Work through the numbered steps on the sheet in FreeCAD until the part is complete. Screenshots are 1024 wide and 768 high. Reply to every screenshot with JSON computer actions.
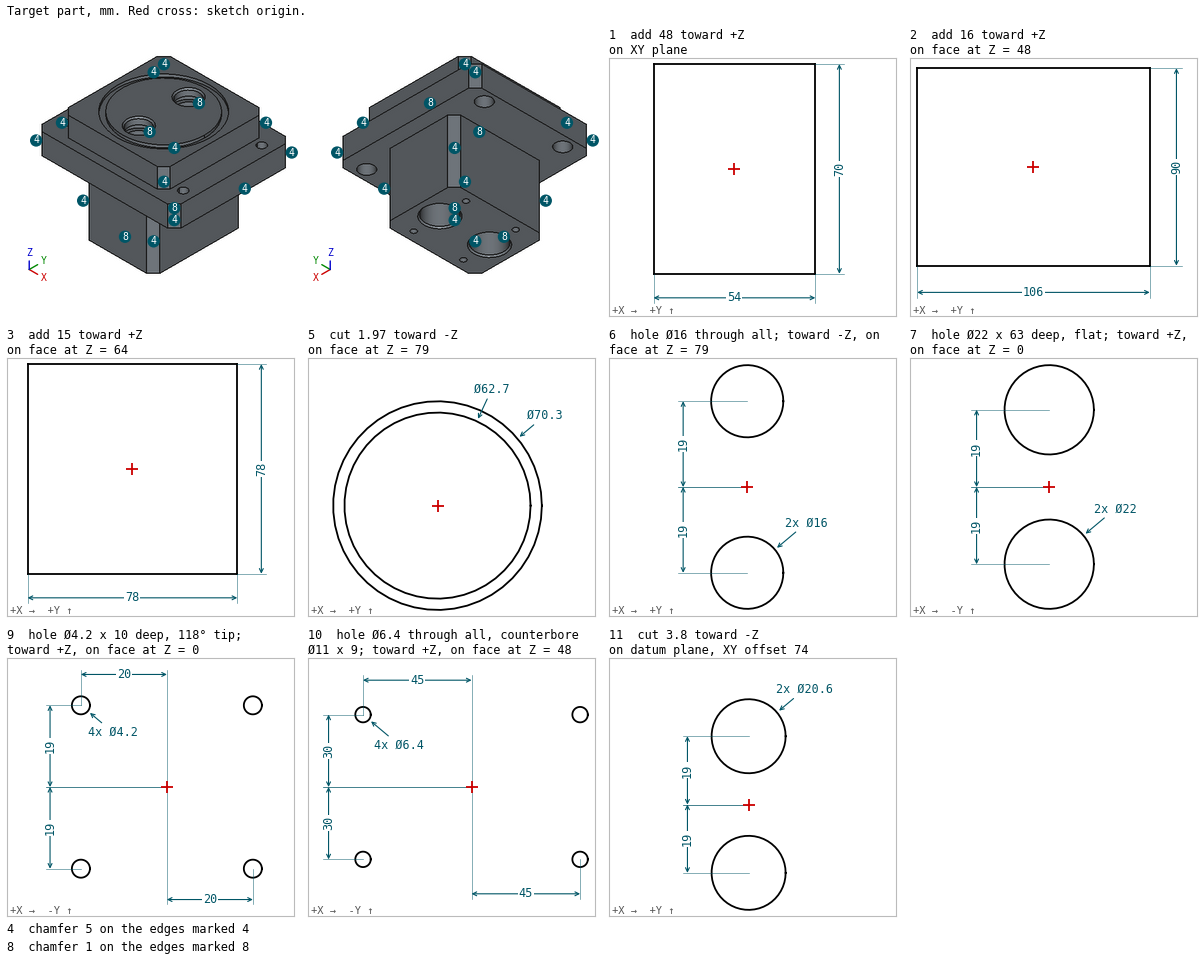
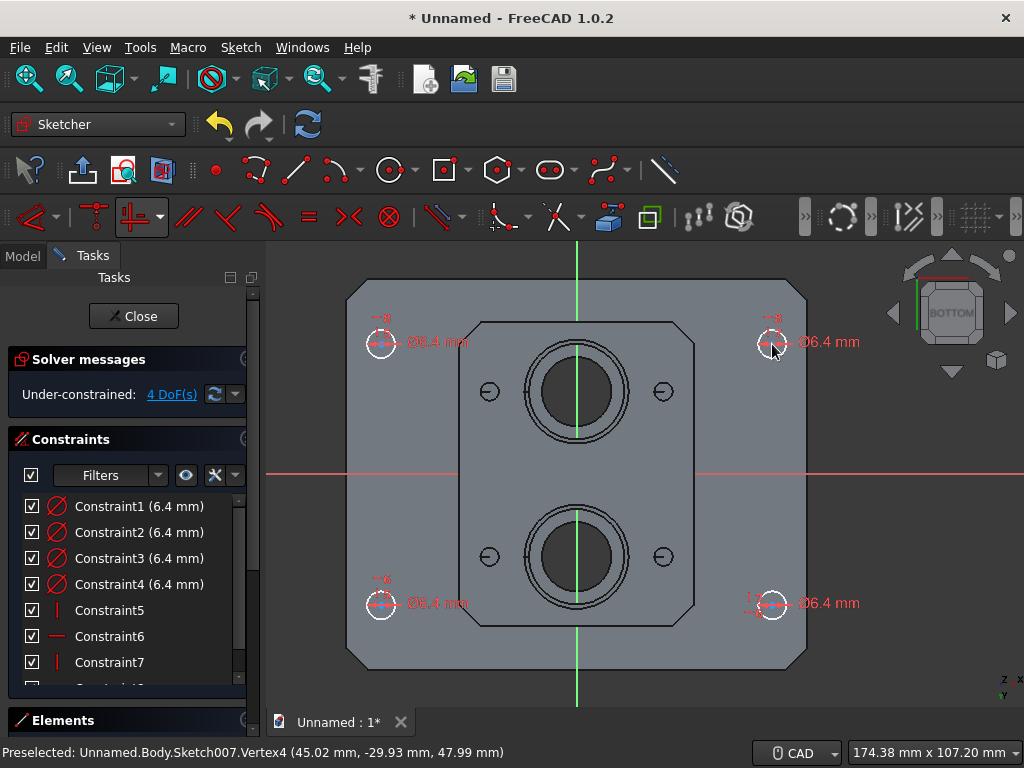
{"action": "left_click", "coordinate": [32, 218]}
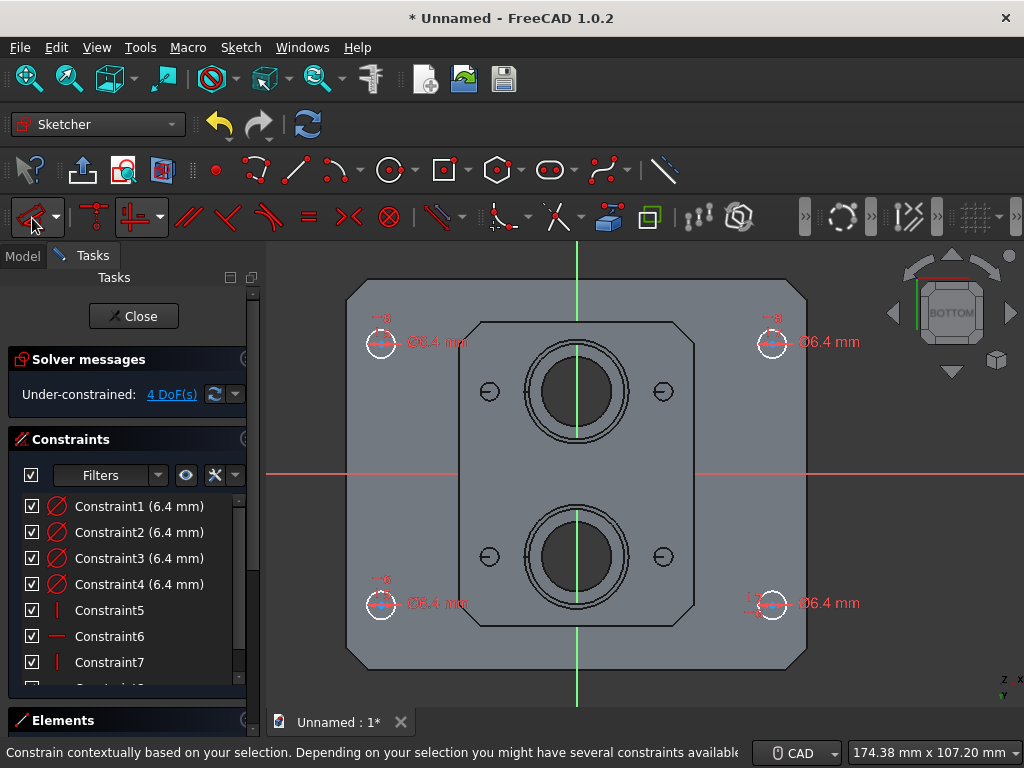
{"action": "left_click", "coordinate": [381, 344]}
{"action": "left_click", "coordinate": [479, 310]}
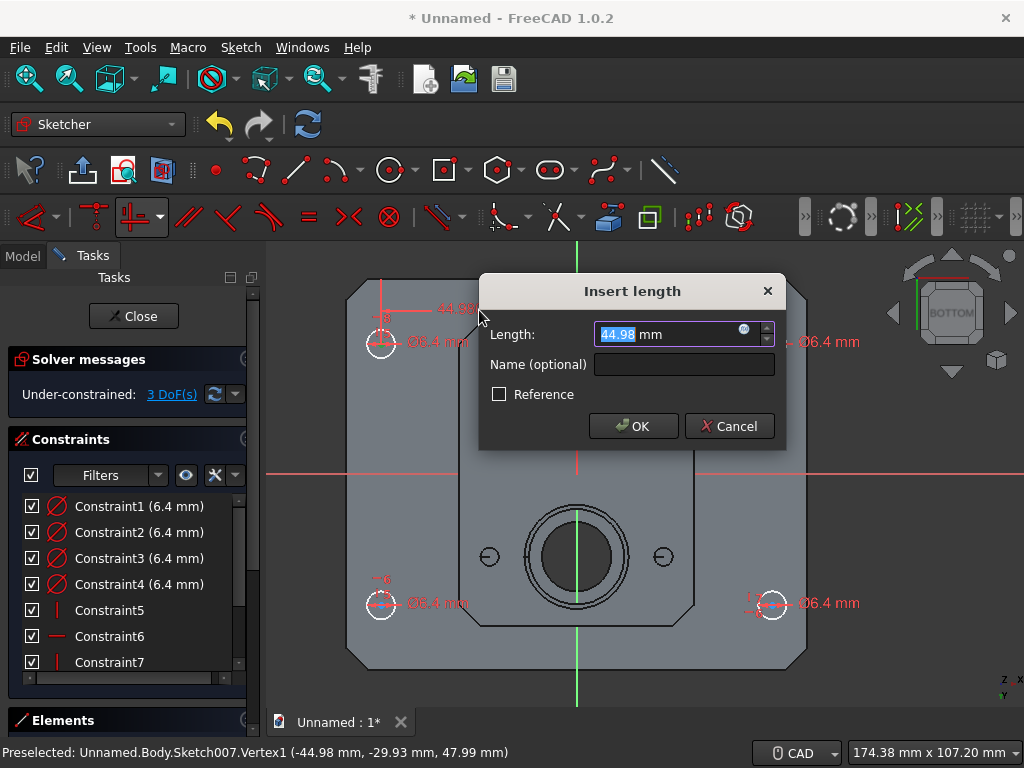
{"action": "type", "text": "45"}
{"action": "key", "text": "Return"}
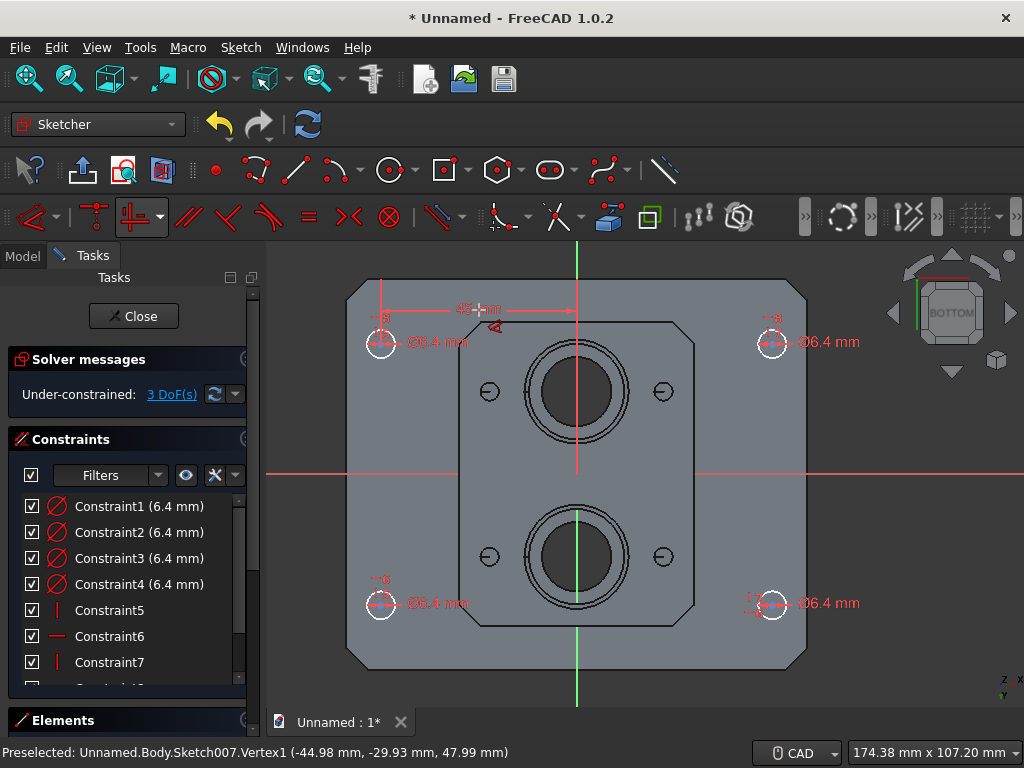
{"action": "left_click", "coordinate": [381, 344]}
{"action": "left_click", "coordinate": [347, 409]}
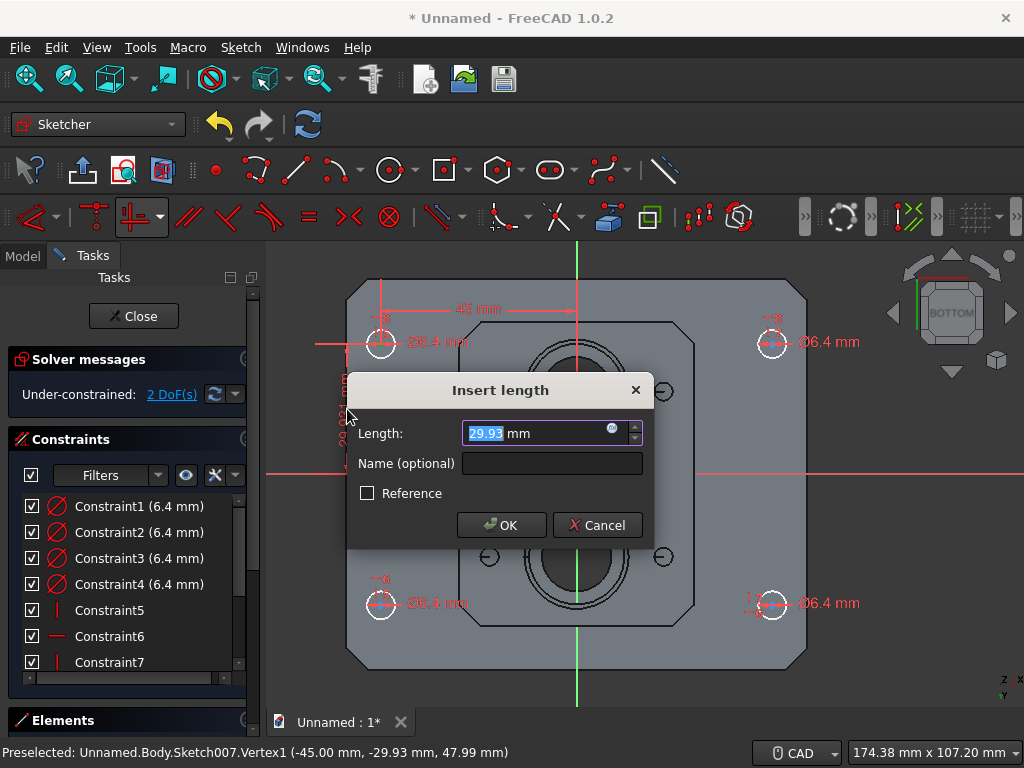
{"action": "type", "text": "30"}
{"action": "key", "text": "Return"}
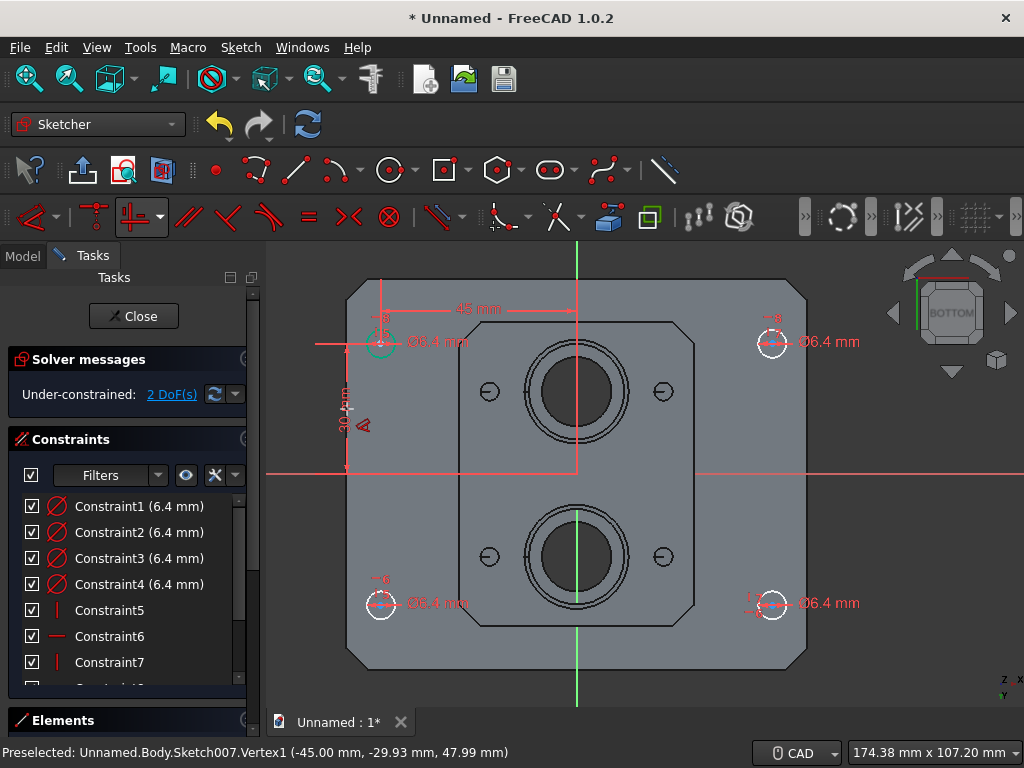
{"action": "left_click", "coordinate": [381, 605]}
{"action": "left_click", "coordinate": [347, 540]}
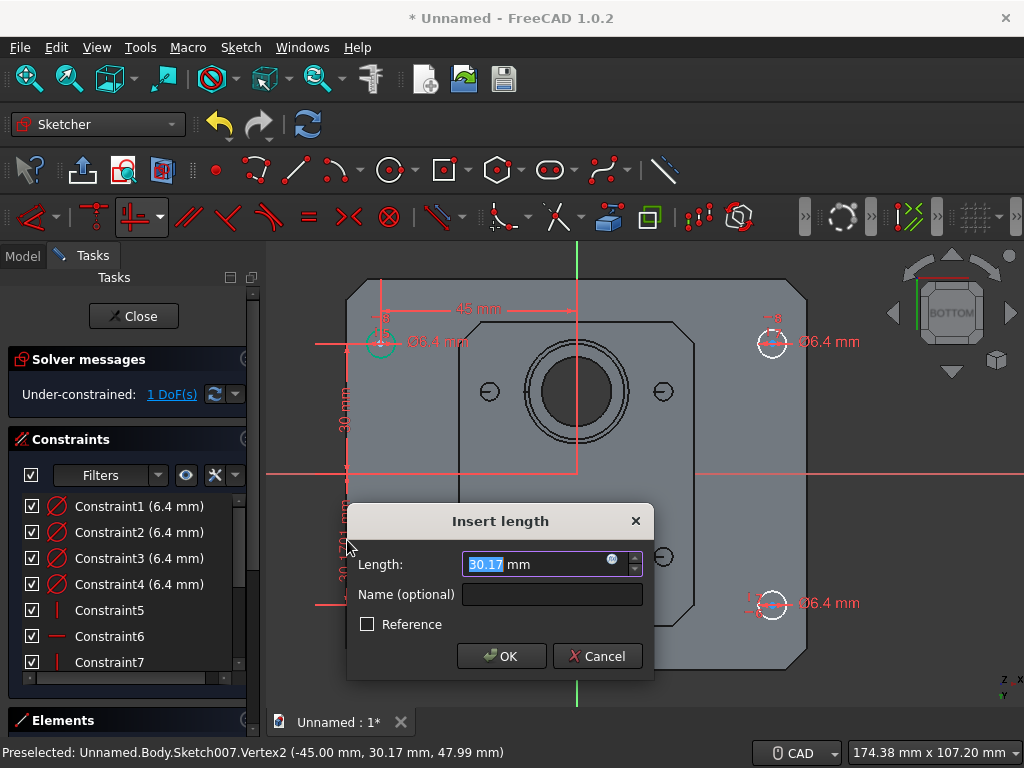
{"action": "type", "text": "30"}
{"action": "key", "text": "Return"}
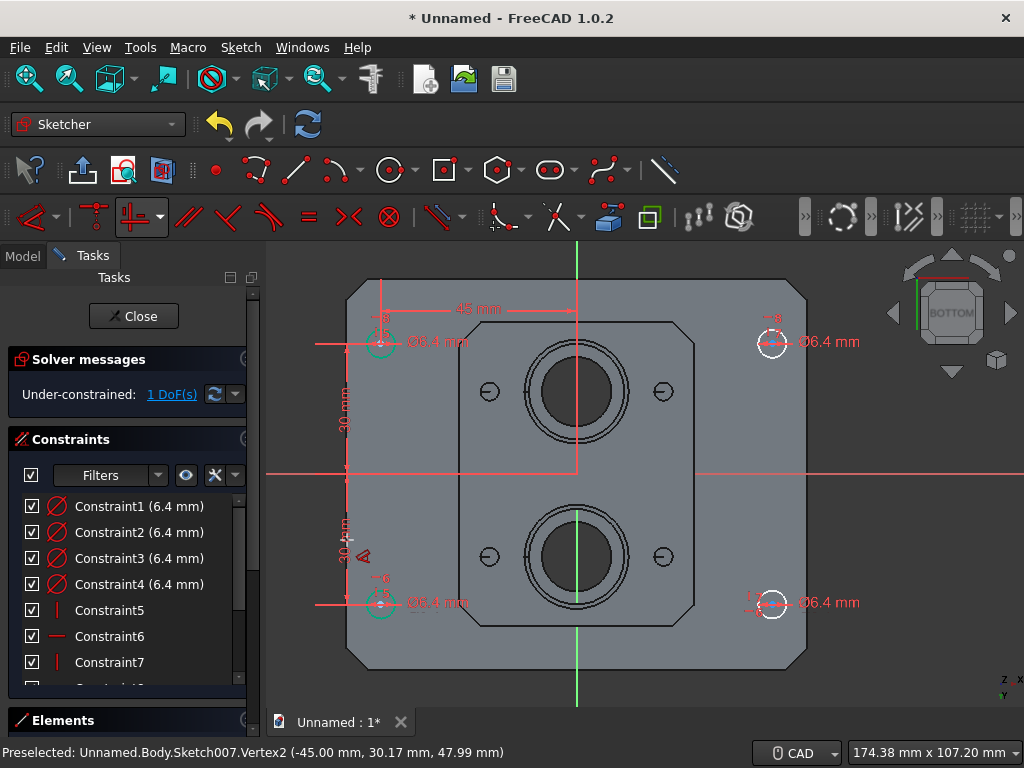
{"action": "left_click", "coordinate": [772, 605]}
{"action": "left_click", "coordinate": [674, 639]}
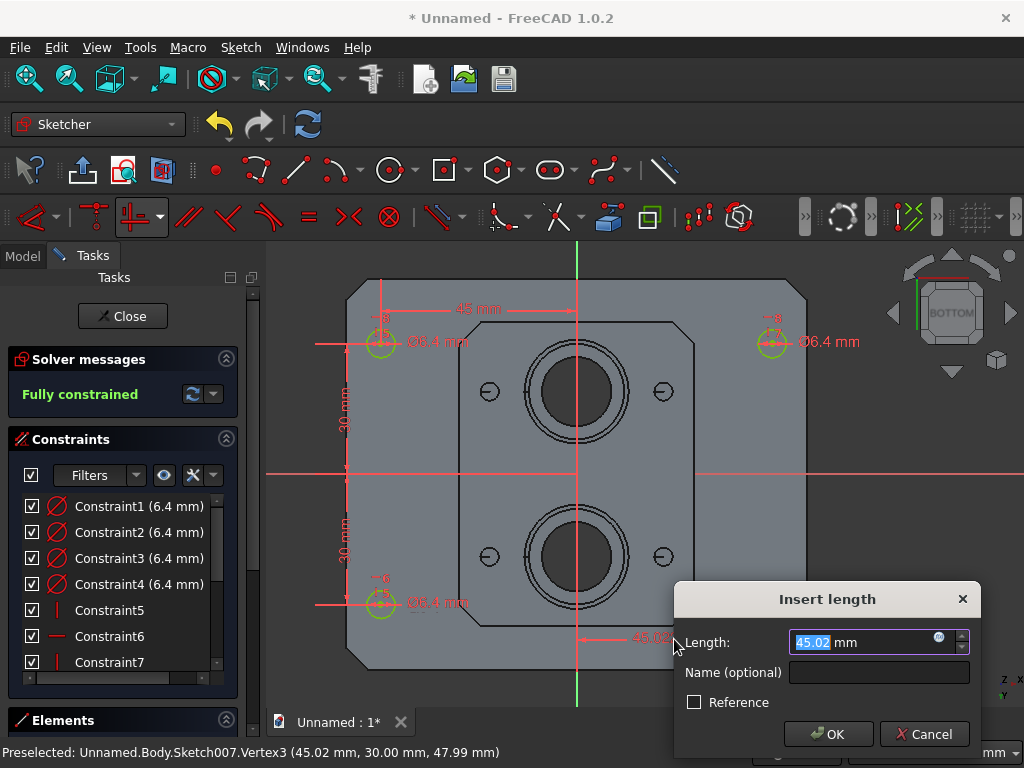
{"action": "type", "text": "45"}
{"action": "key", "text": "Return"}
{"action": "key", "text": "Escape"}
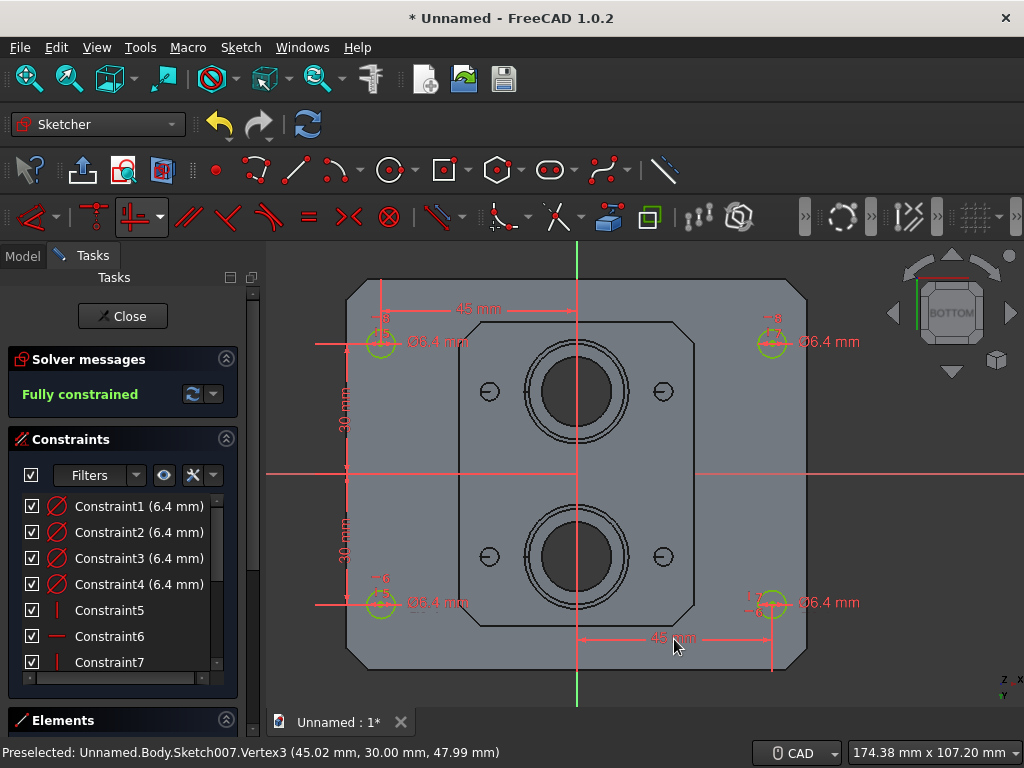
{"action": "left_click", "coordinate": [123, 316]}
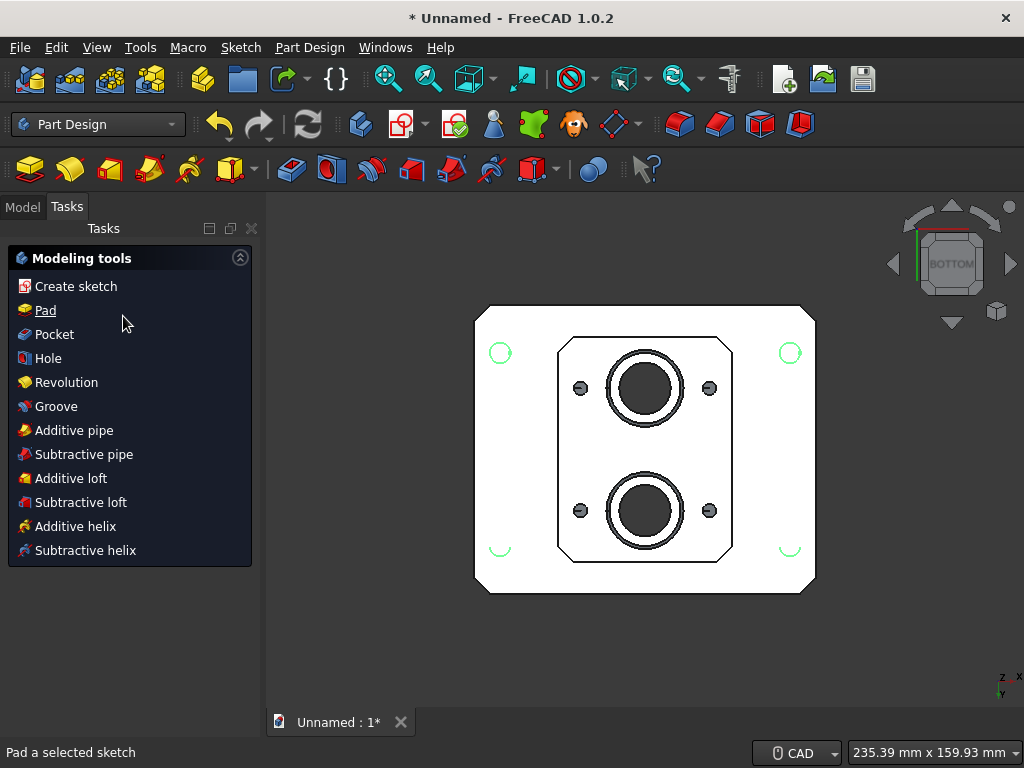
{"action": "left_click", "coordinate": [332, 170]}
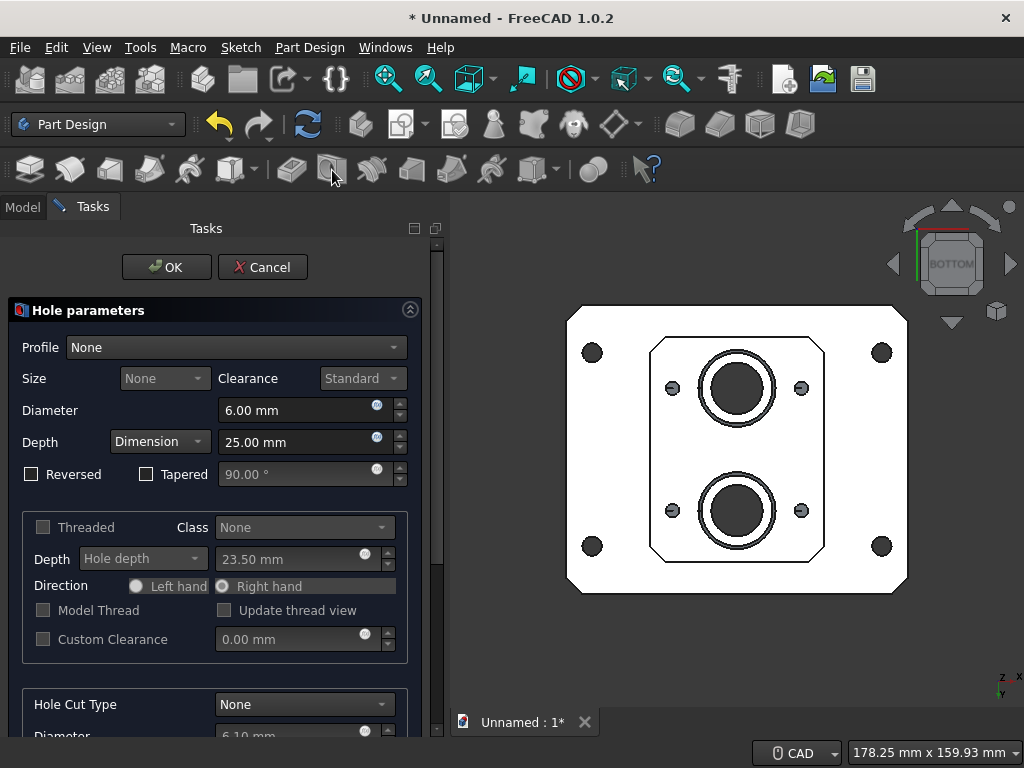
{"action": "triple_click", "coordinate": [305, 410]}